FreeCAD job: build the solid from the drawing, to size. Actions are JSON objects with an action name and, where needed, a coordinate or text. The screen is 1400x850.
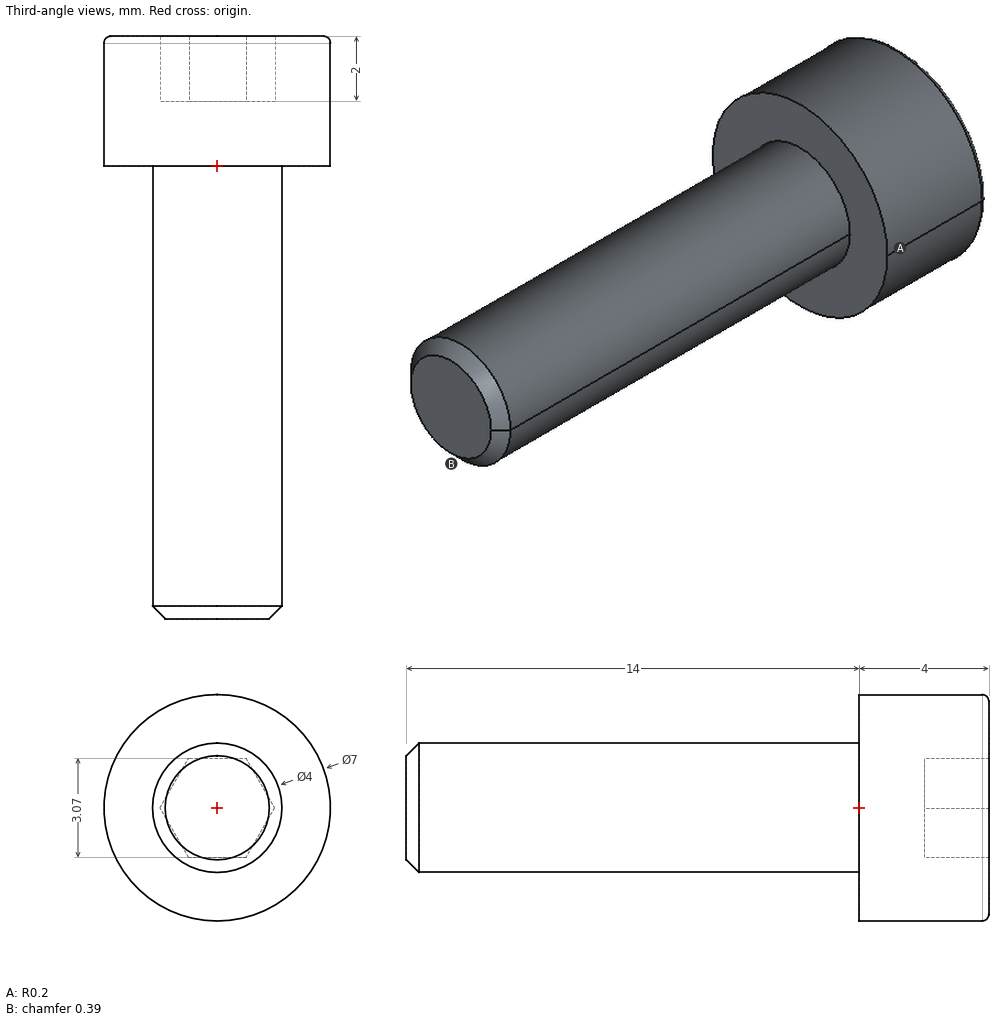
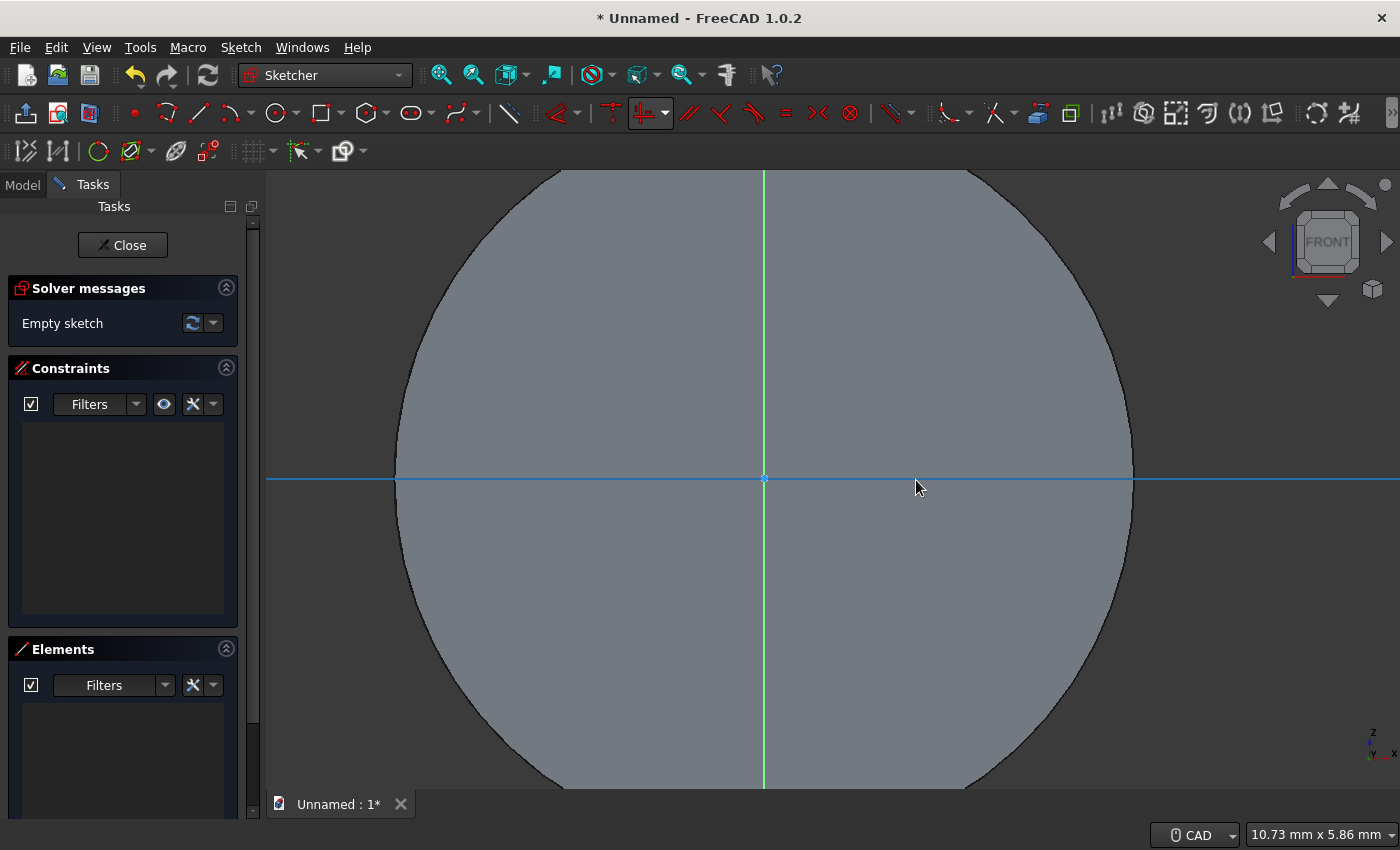
{"action": "left_click", "coordinate": [276, 114]}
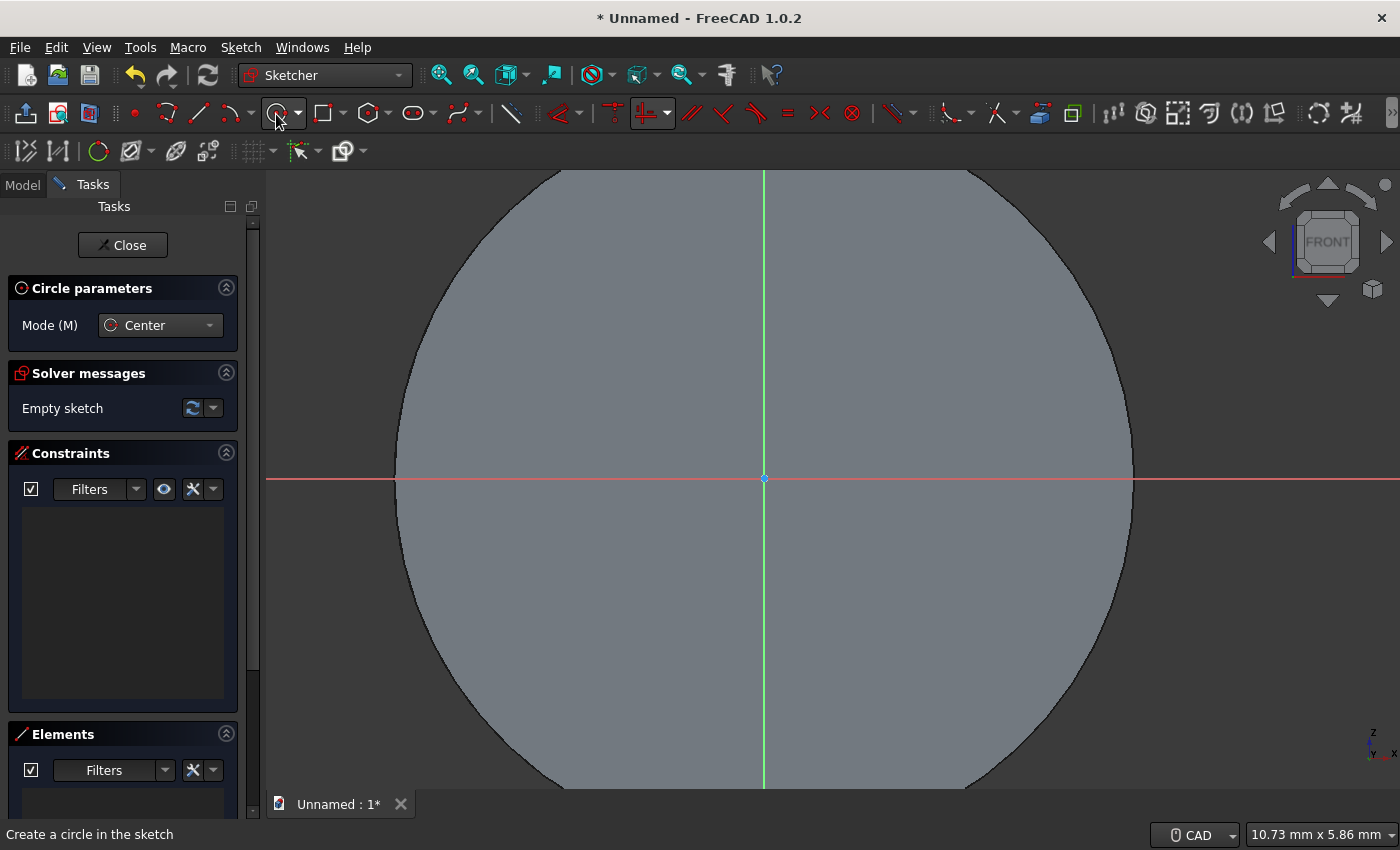
{"action": "left_click", "coordinate": [764, 479]}
{"action": "mouse_move", "coordinate": [914, 329]}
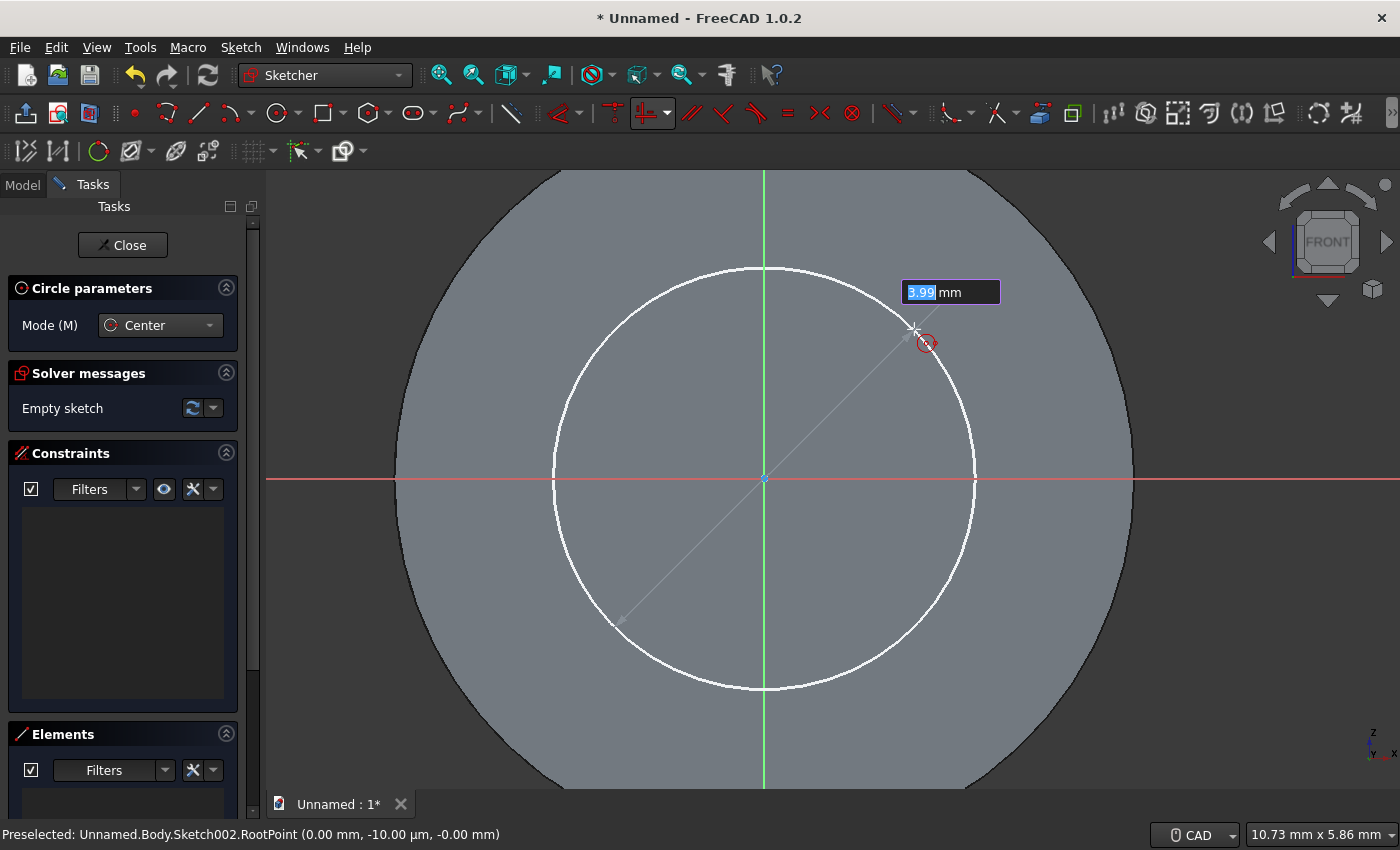
{"action": "type", "text": "4"}
{"action": "key", "text": "Return"}
{"action": "key", "text": "Escape"}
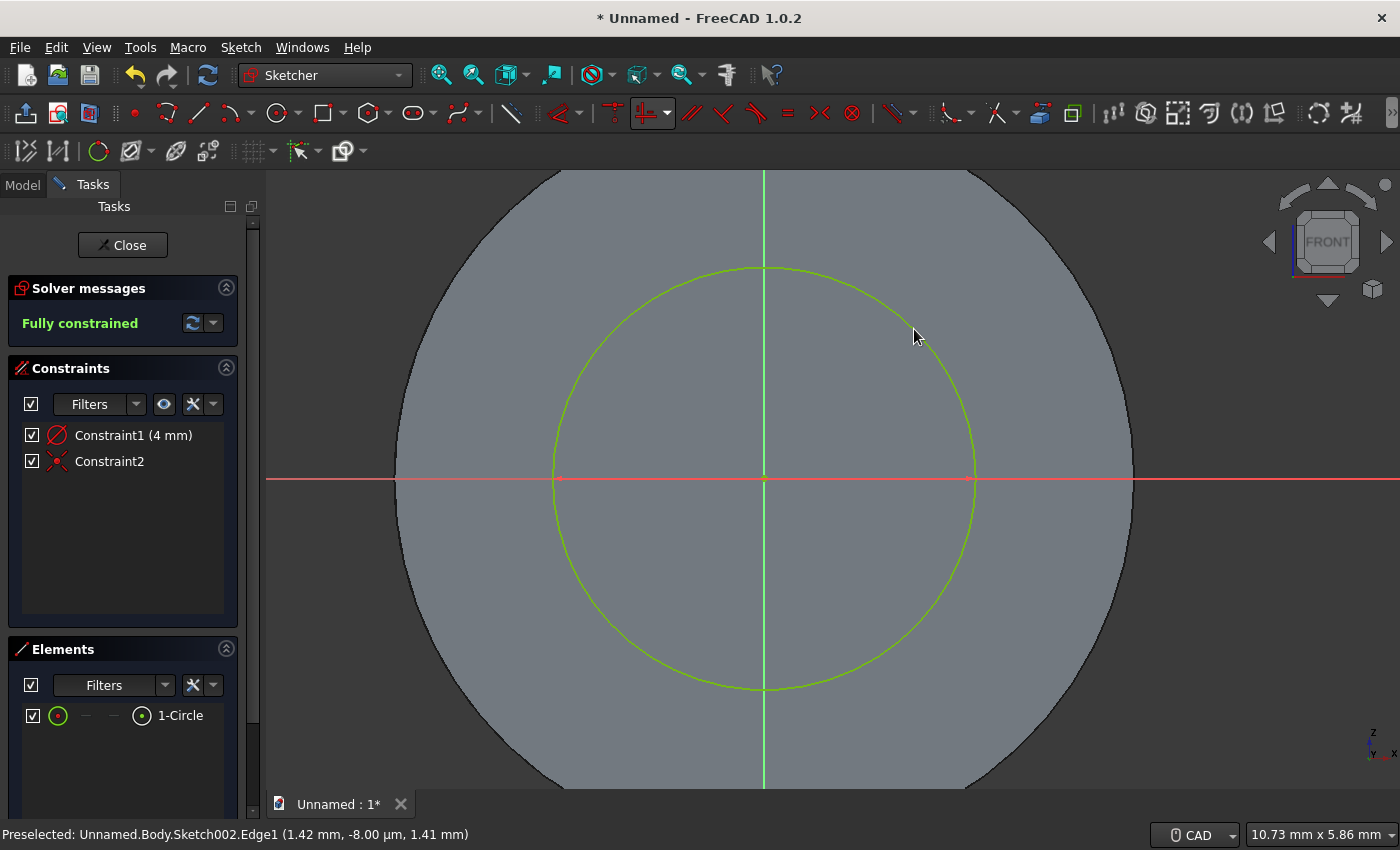
{"action": "left_click", "coordinate": [123, 245]}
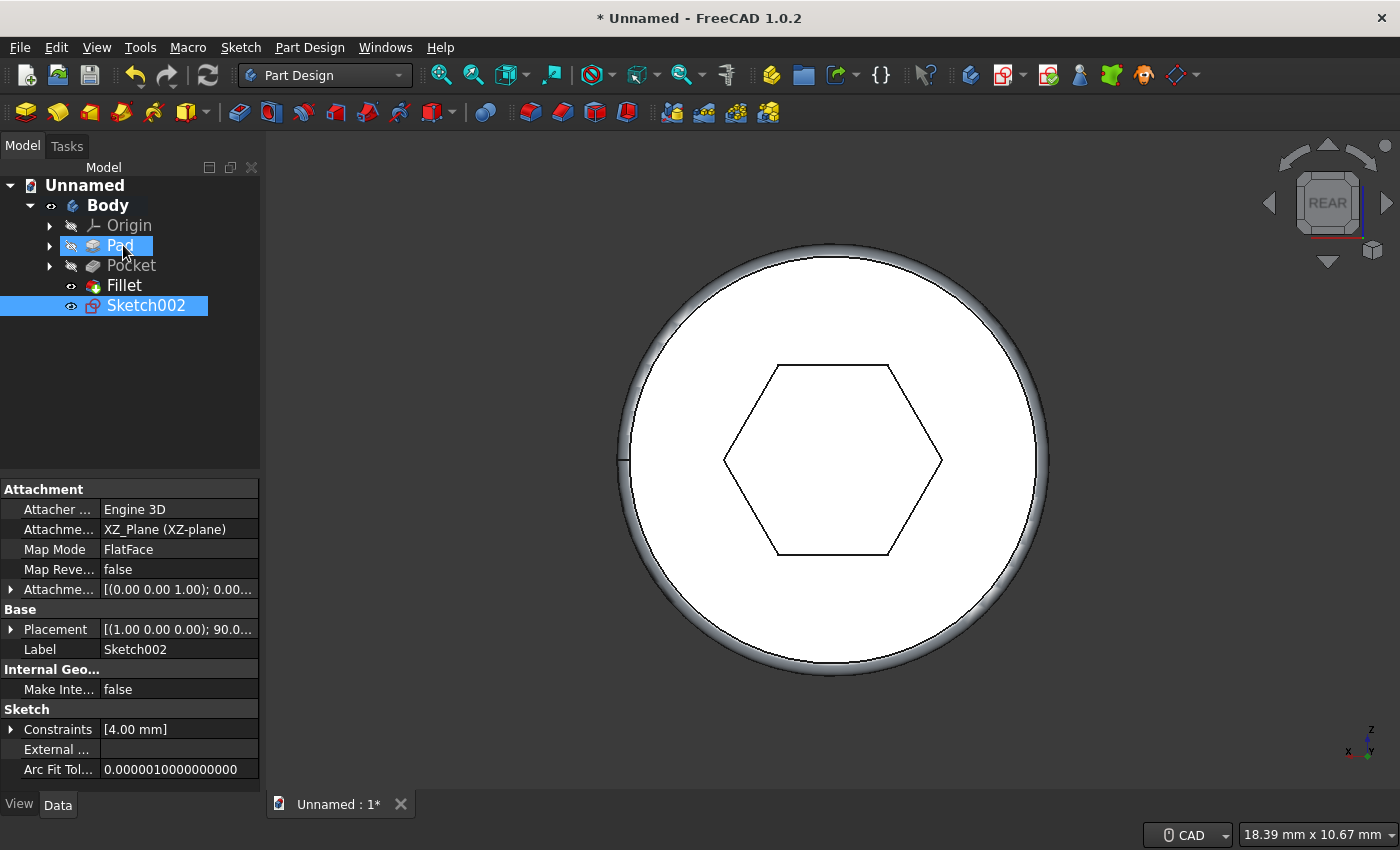
{"action": "left_click", "coordinate": [26, 112]}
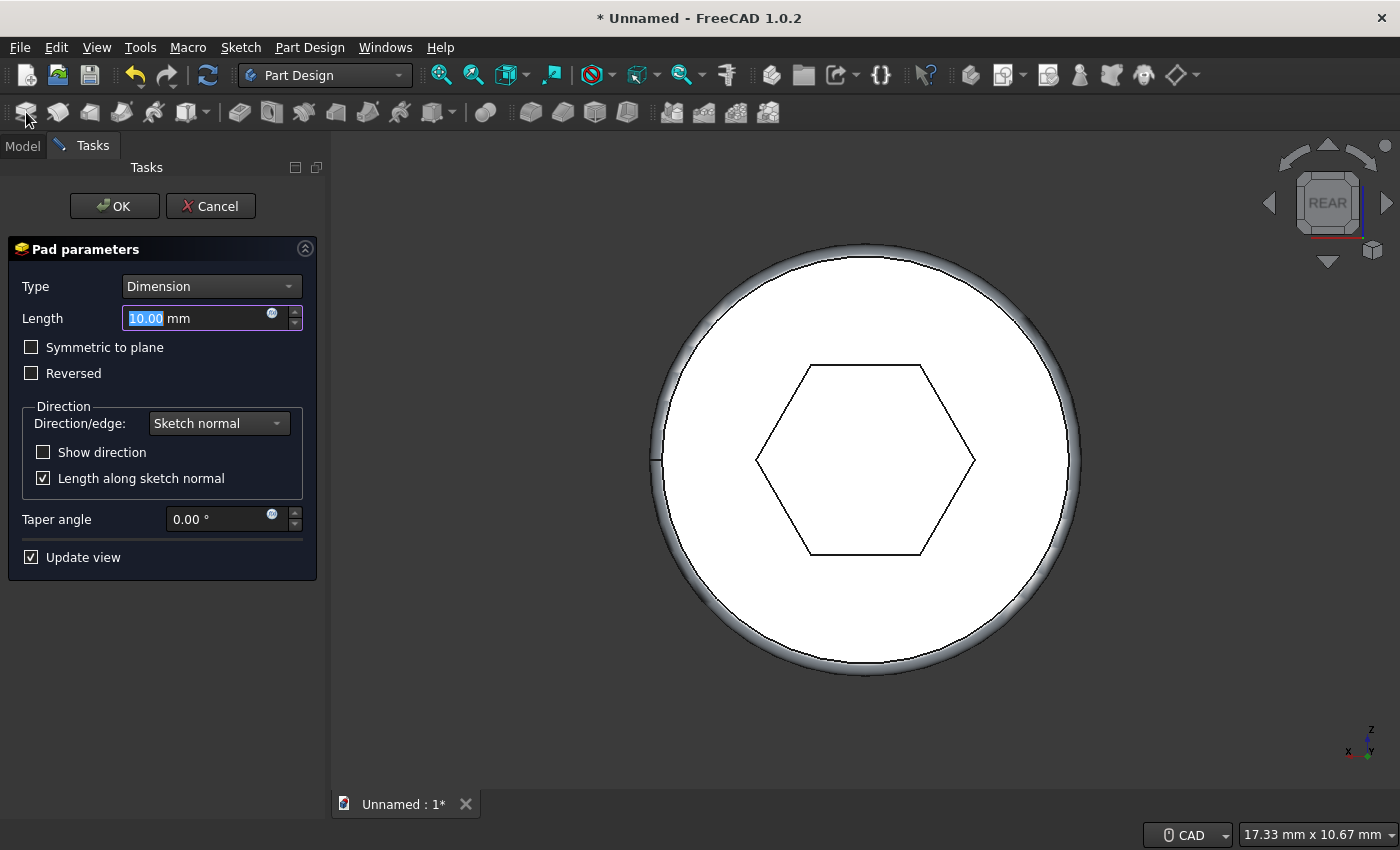
{"action": "type", "text": "14"}
{"action": "key", "text": "Tab"}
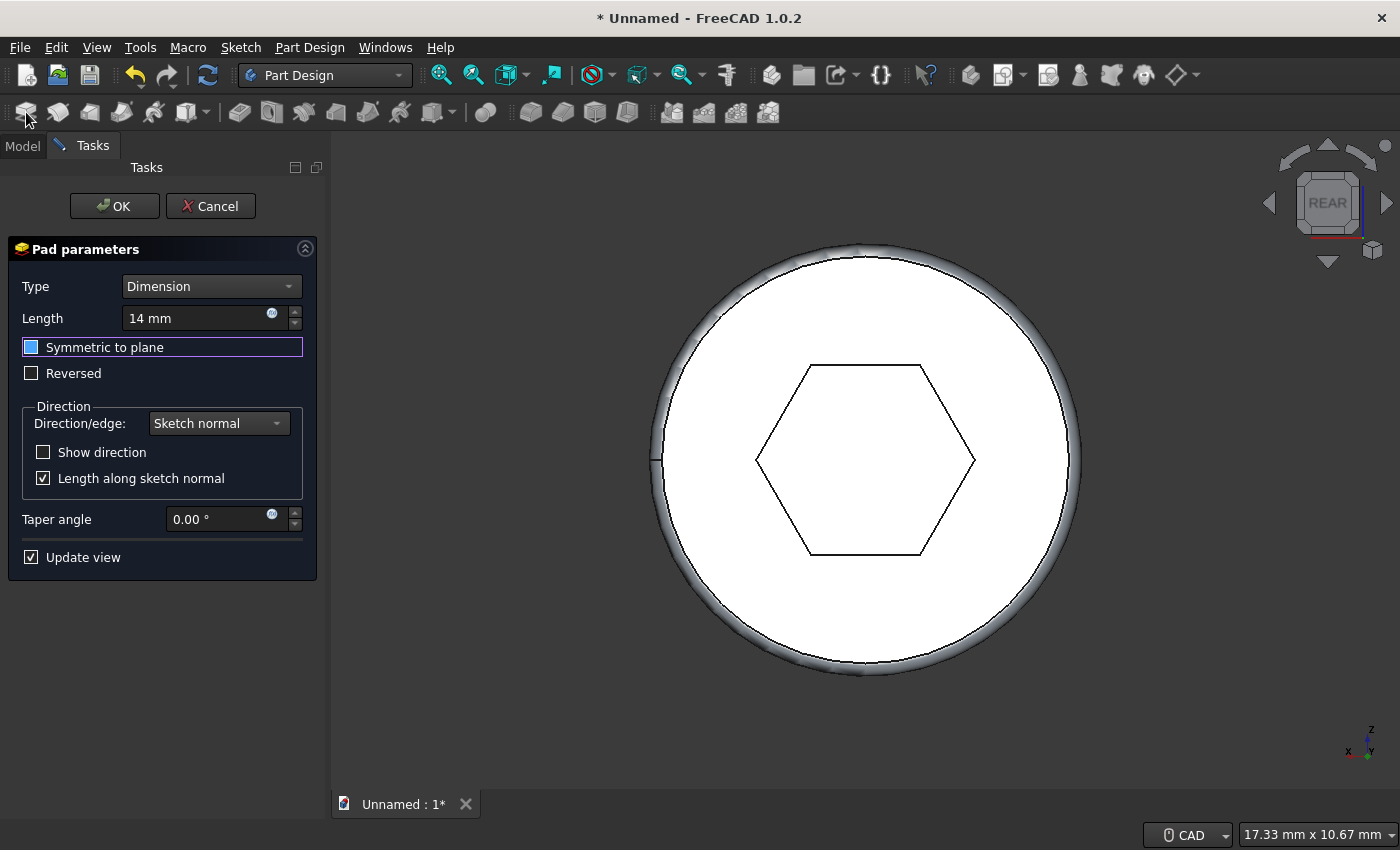
{"action": "left_click", "coordinate": [115, 206]}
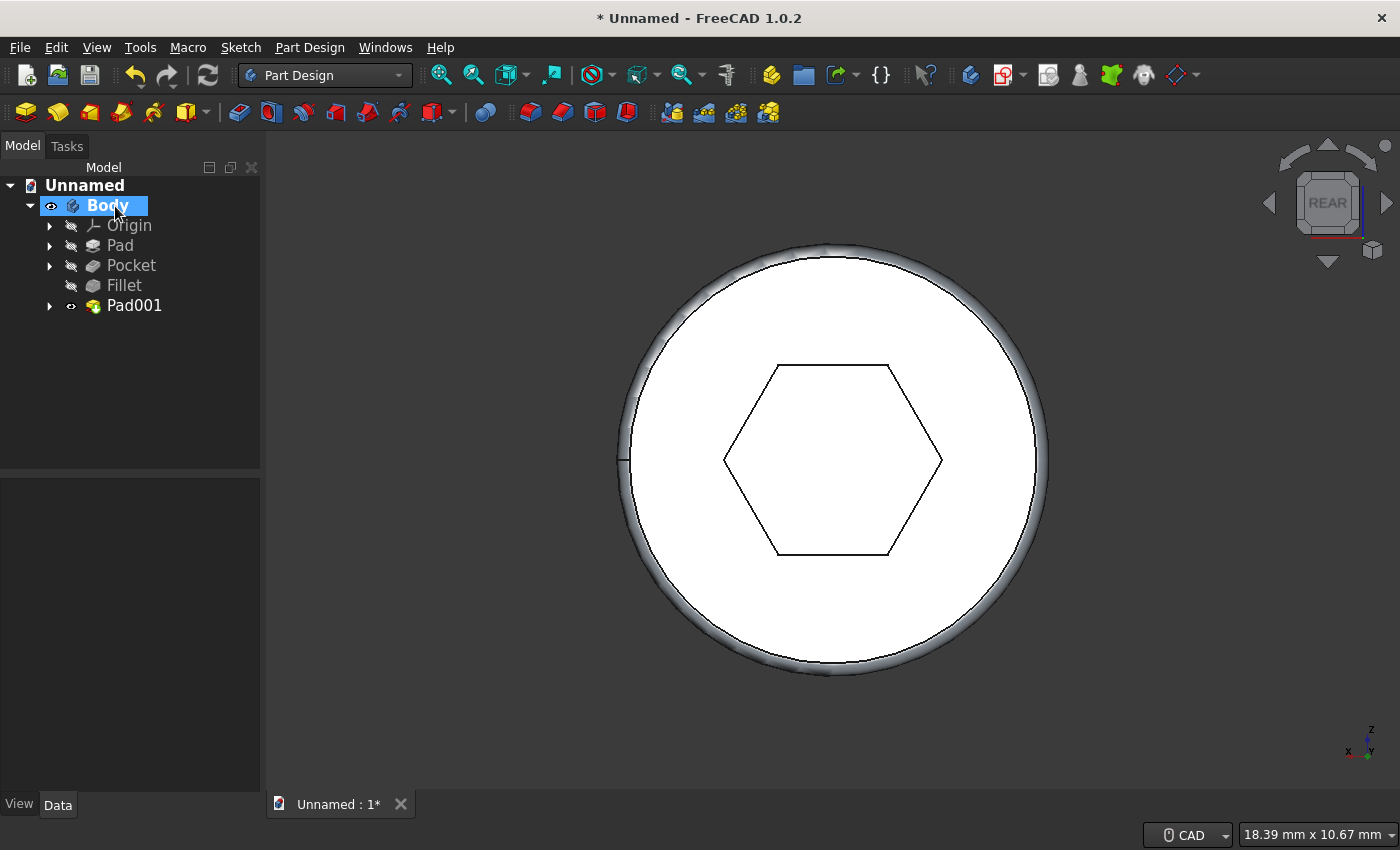
{"action": "key", "text": "0"}